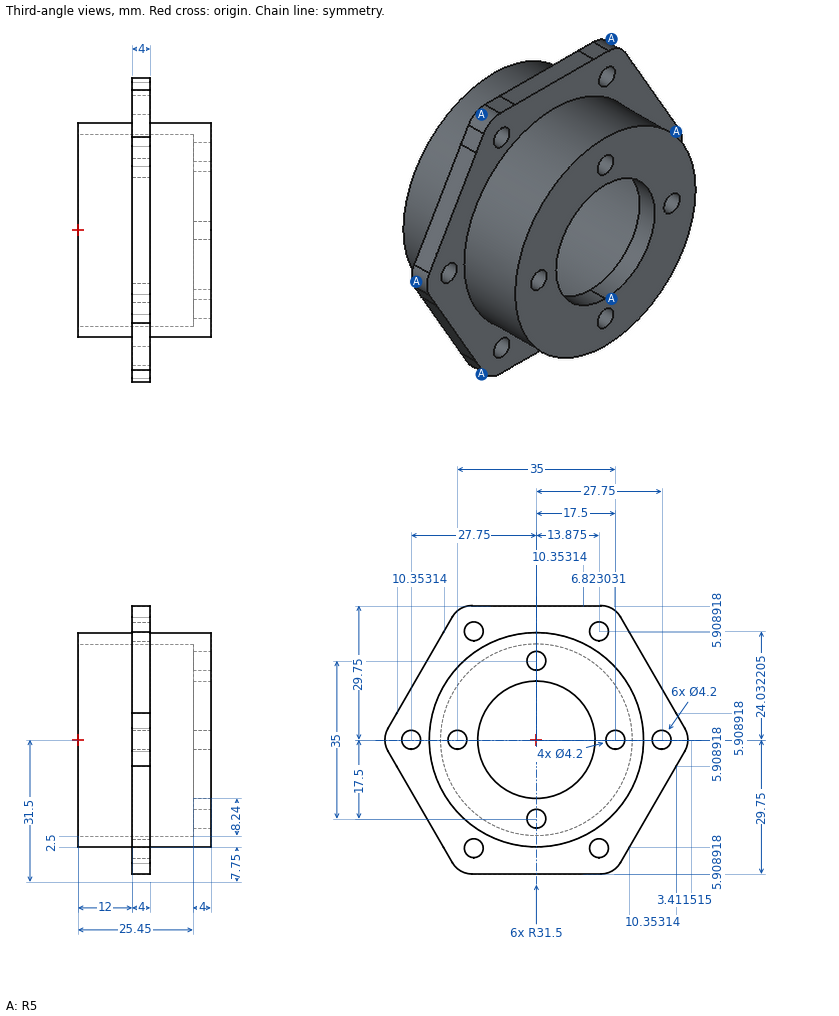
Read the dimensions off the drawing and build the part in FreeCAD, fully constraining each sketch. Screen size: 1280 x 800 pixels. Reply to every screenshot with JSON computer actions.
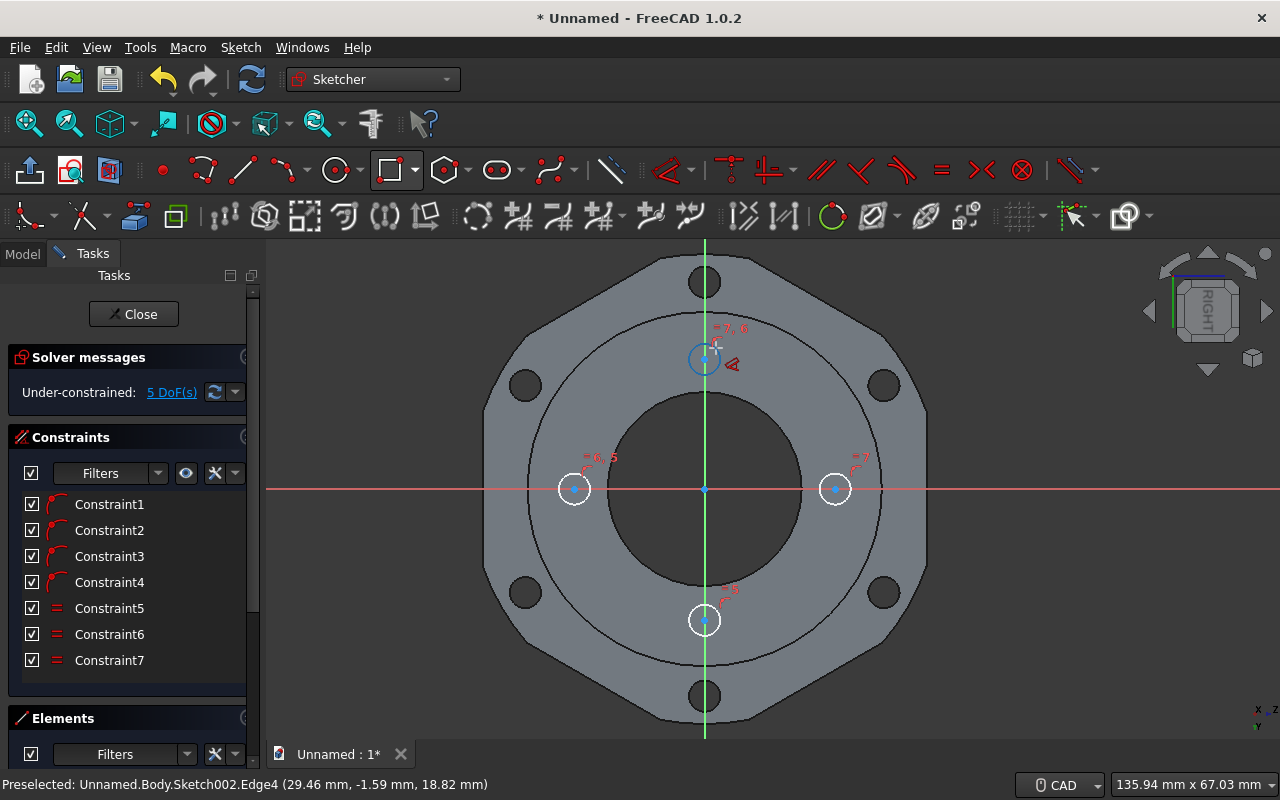
{"action": "scroll", "coordinate": [716, 609], "scroll_direction": "up", "scroll_amount": 2}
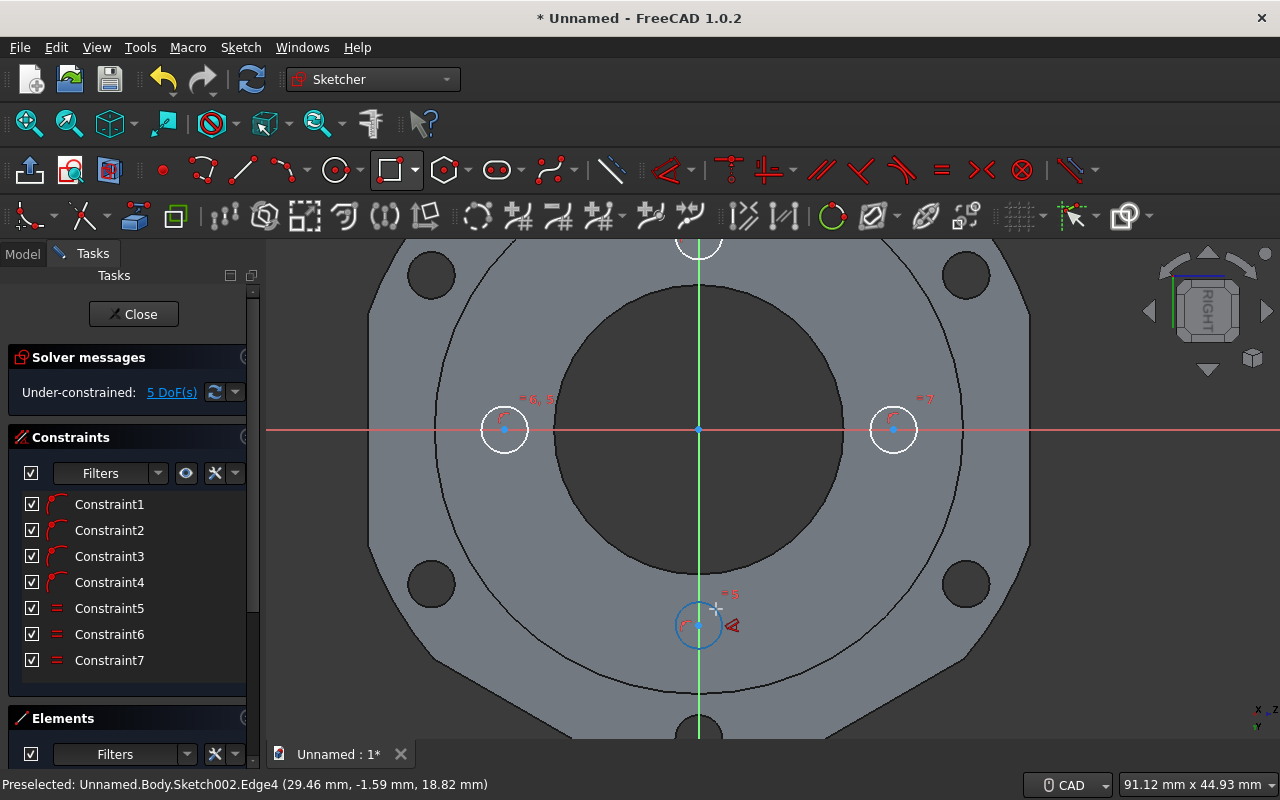
{"action": "left_click", "coordinate": [715, 609]}
{"action": "left_click", "coordinate": [737, 586]}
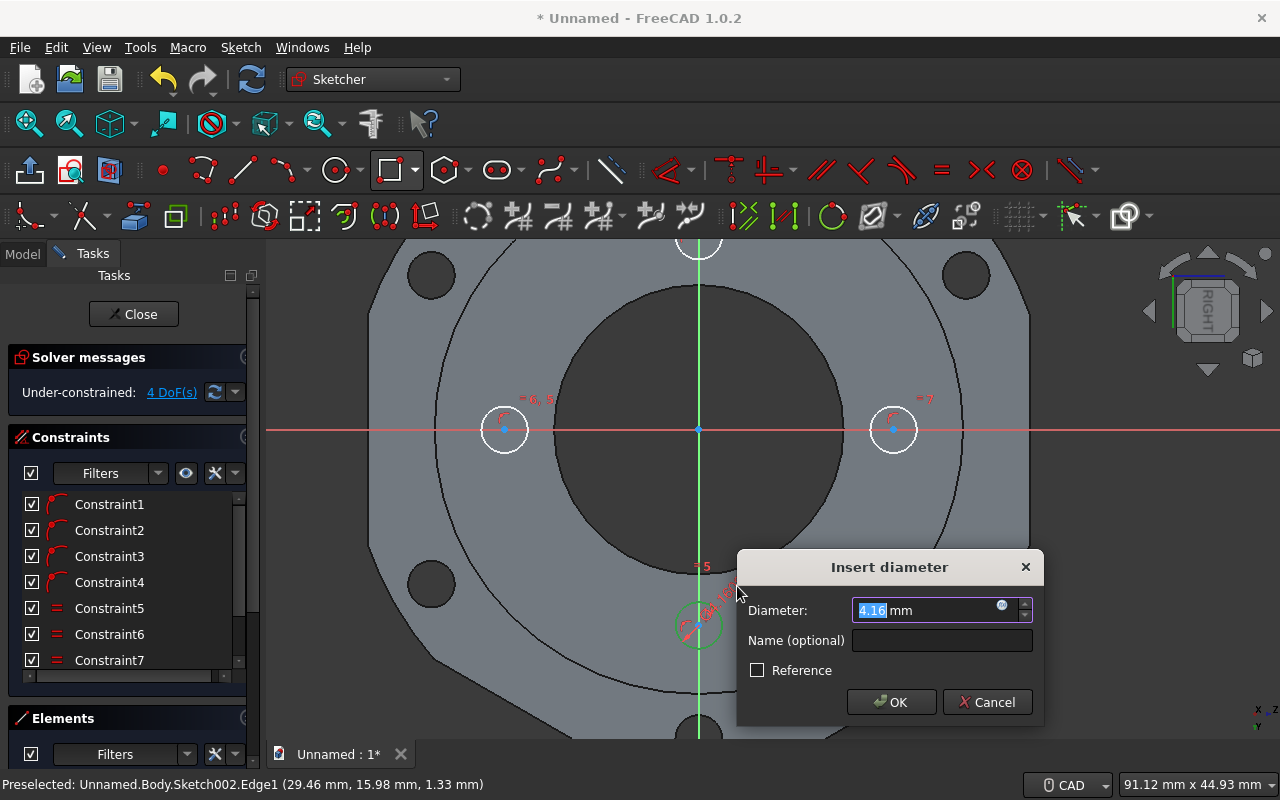
{"action": "type", "text": "4.2"}
{"action": "key", "text": "Return"}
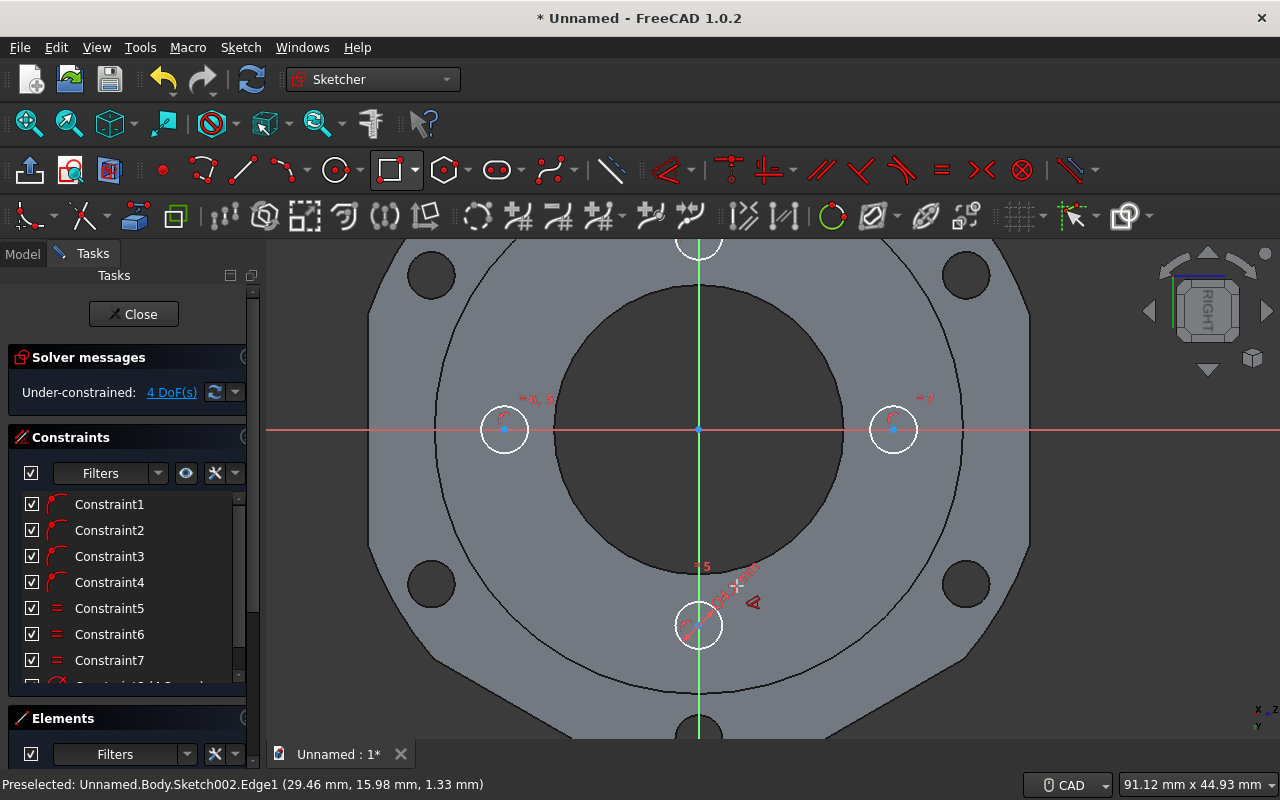
{"action": "left_click", "coordinate": [699, 625]}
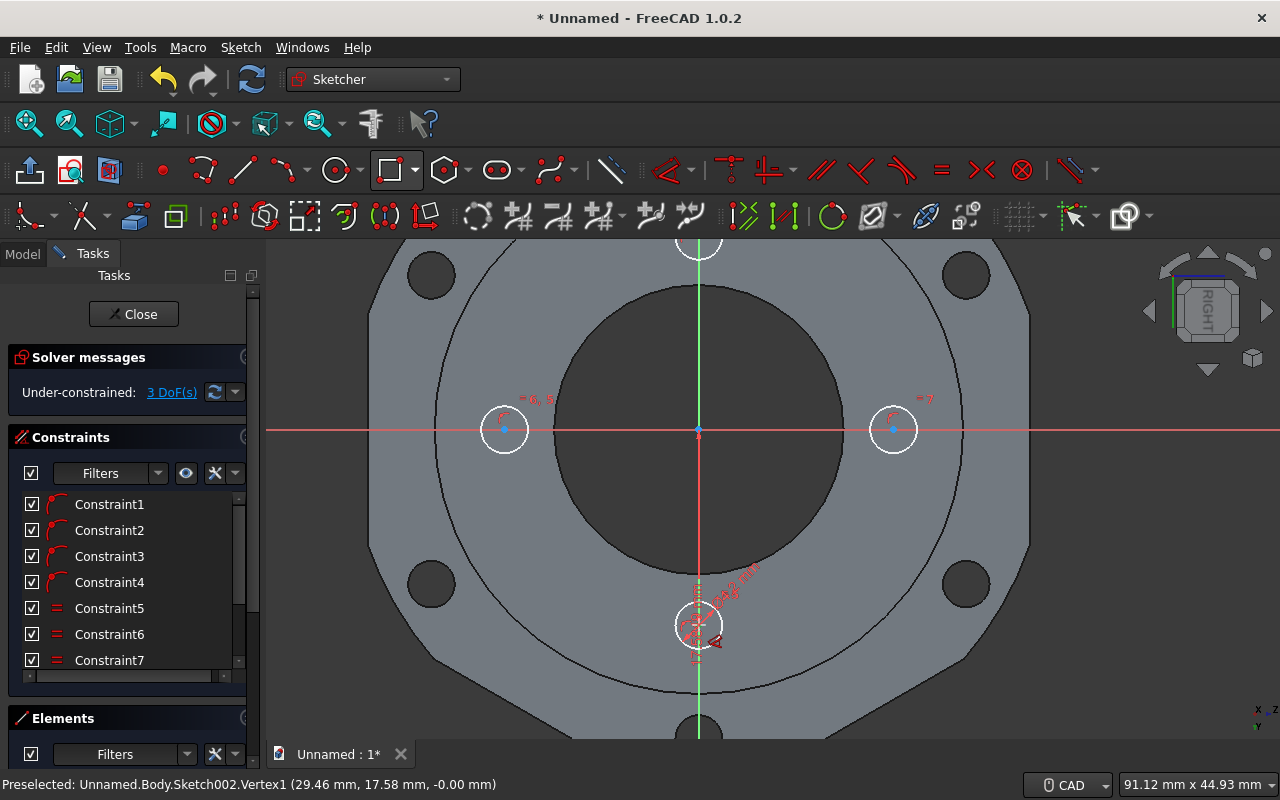
{"action": "scroll", "coordinate": [716, 609], "scroll_direction": "down", "scroll_amount": 2}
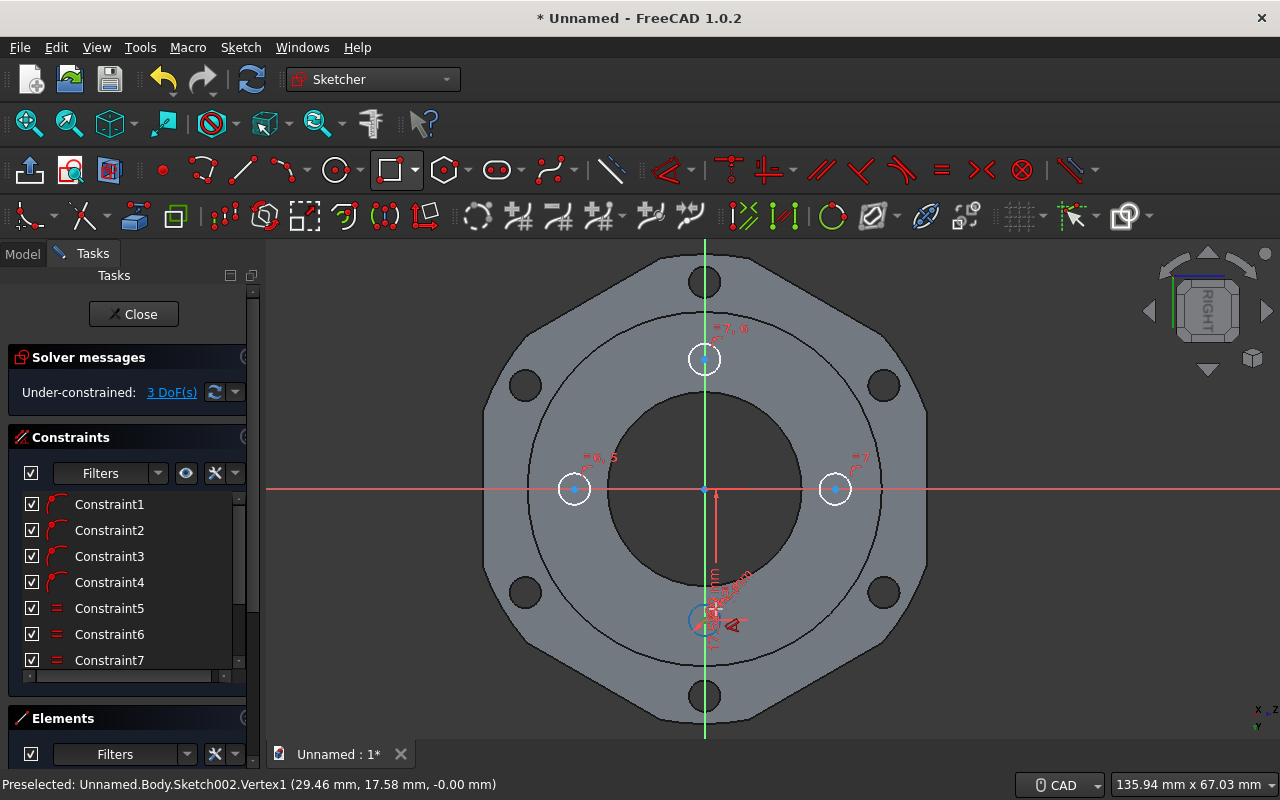
{"action": "left_click", "coordinate": [705, 359]}
{"action": "left_click", "coordinate": [739, 430]}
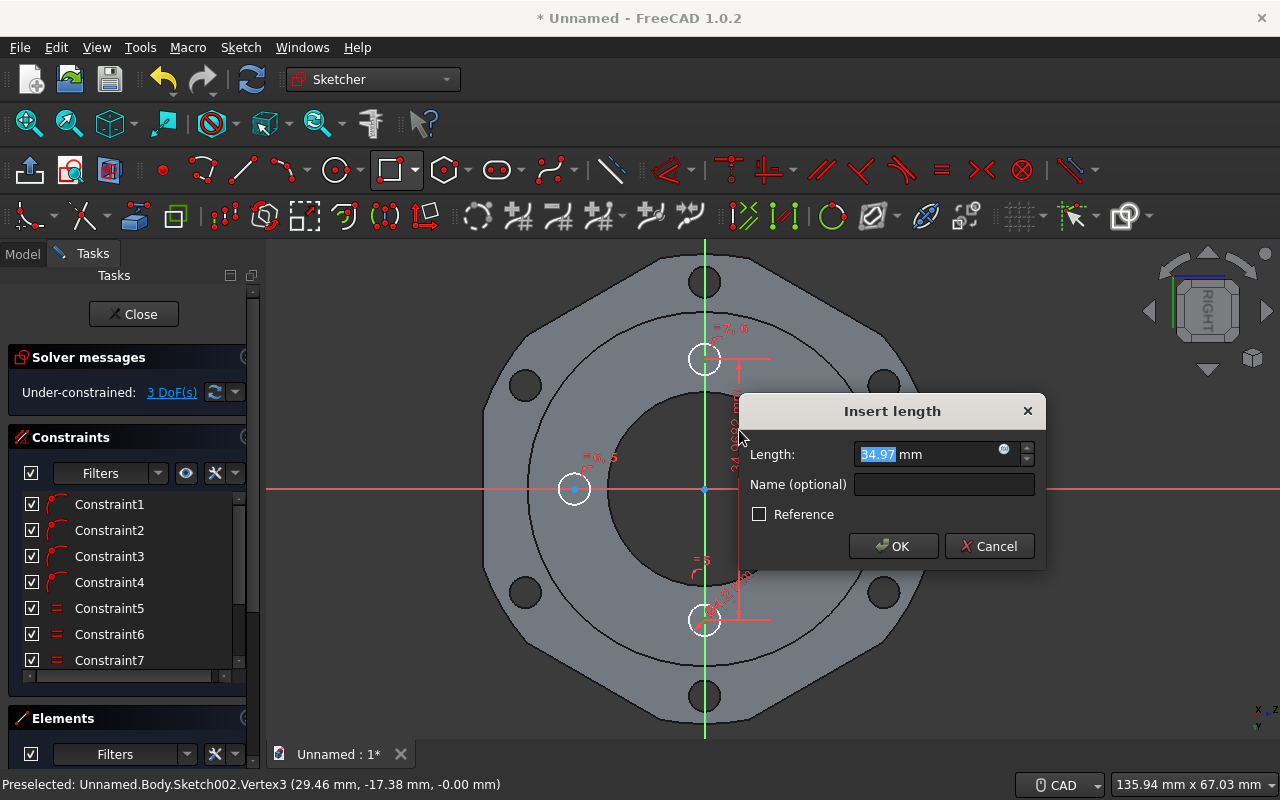
{"action": "type", "text": "35"}
{"action": "key", "text": "Return"}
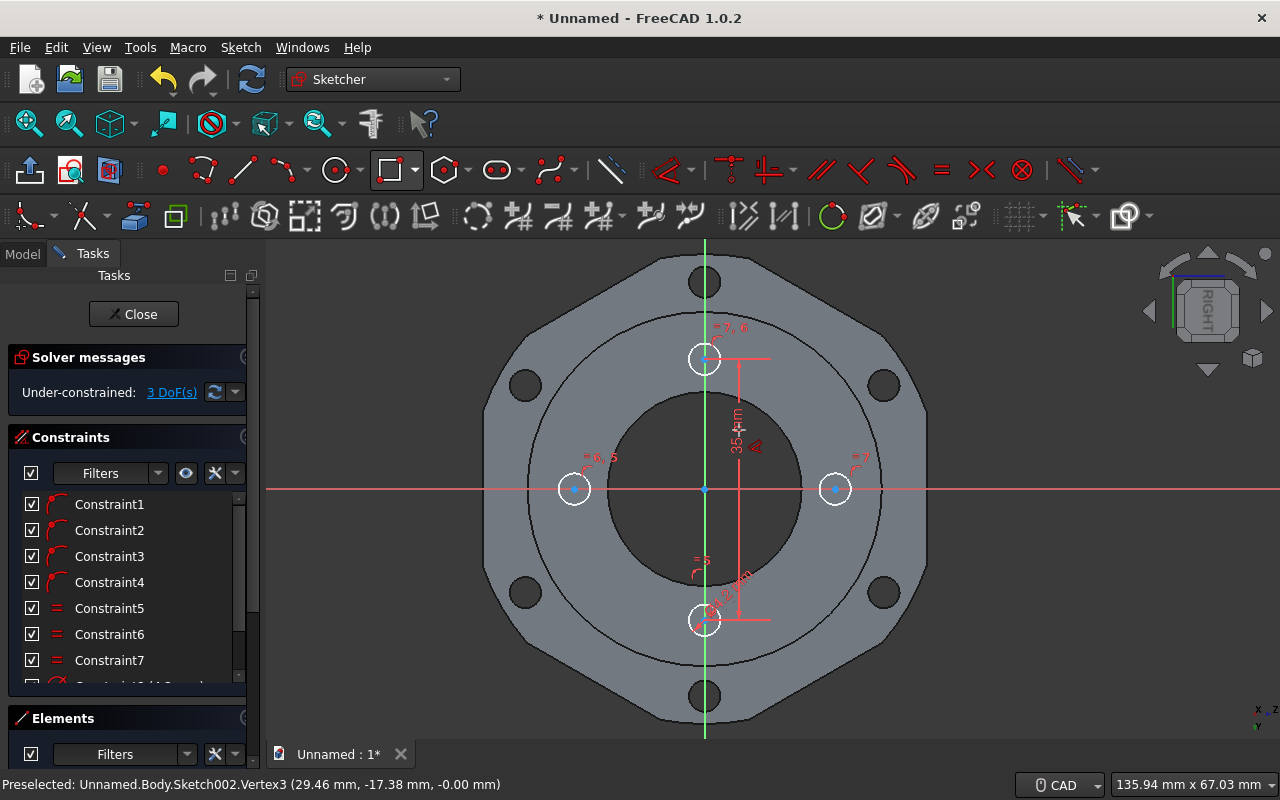
{"action": "left_click", "coordinate": [574, 489]}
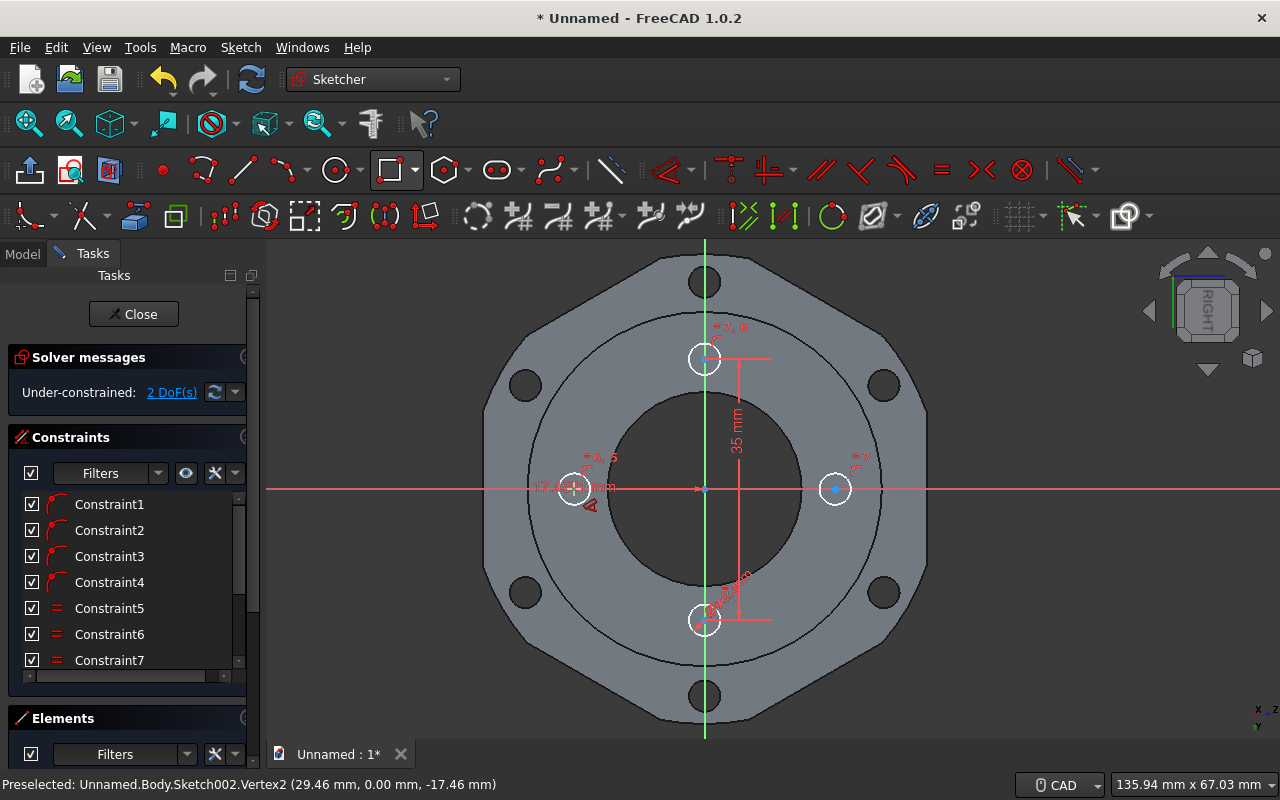
{"action": "left_click", "coordinate": [835, 489]}
{"action": "left_click", "coordinate": [645, 523]}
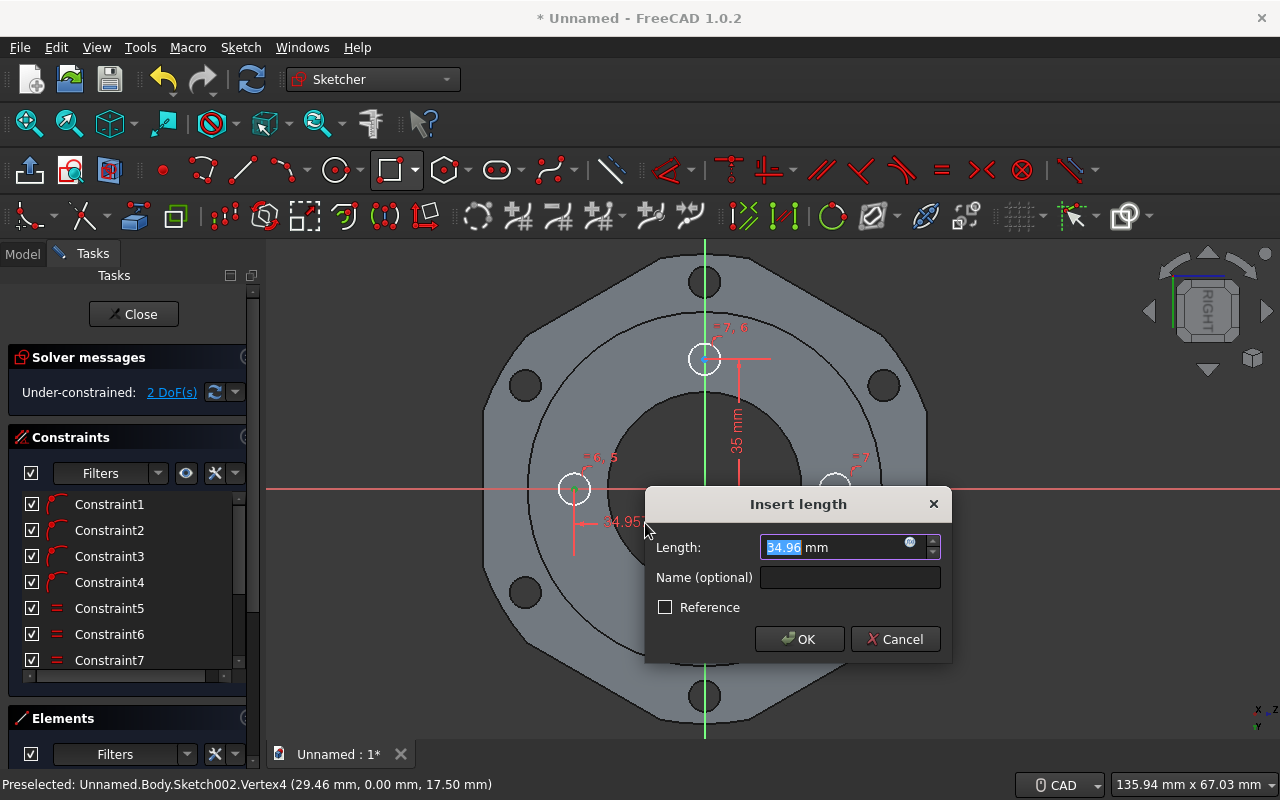
{"action": "type", "text": "35"}
{"action": "key", "text": "Return"}